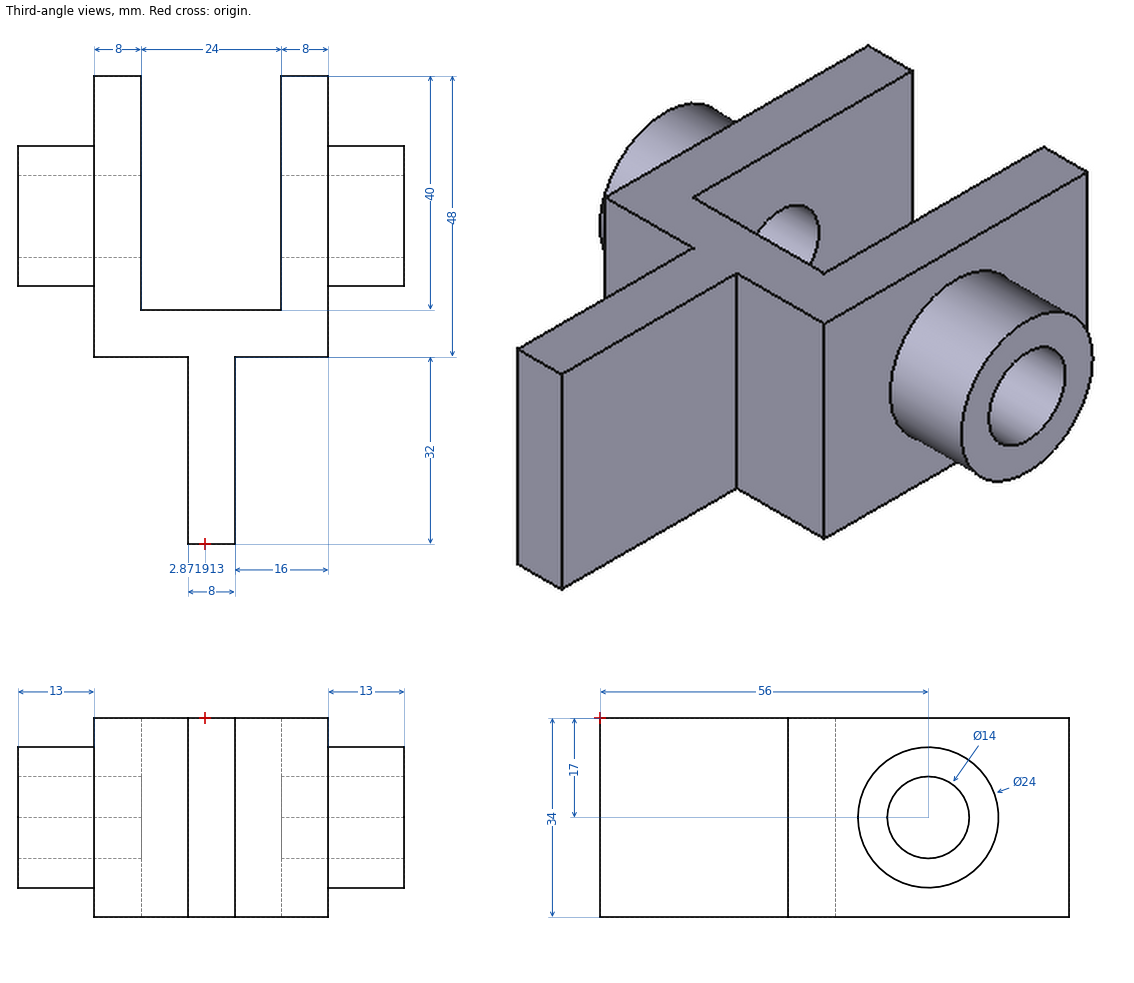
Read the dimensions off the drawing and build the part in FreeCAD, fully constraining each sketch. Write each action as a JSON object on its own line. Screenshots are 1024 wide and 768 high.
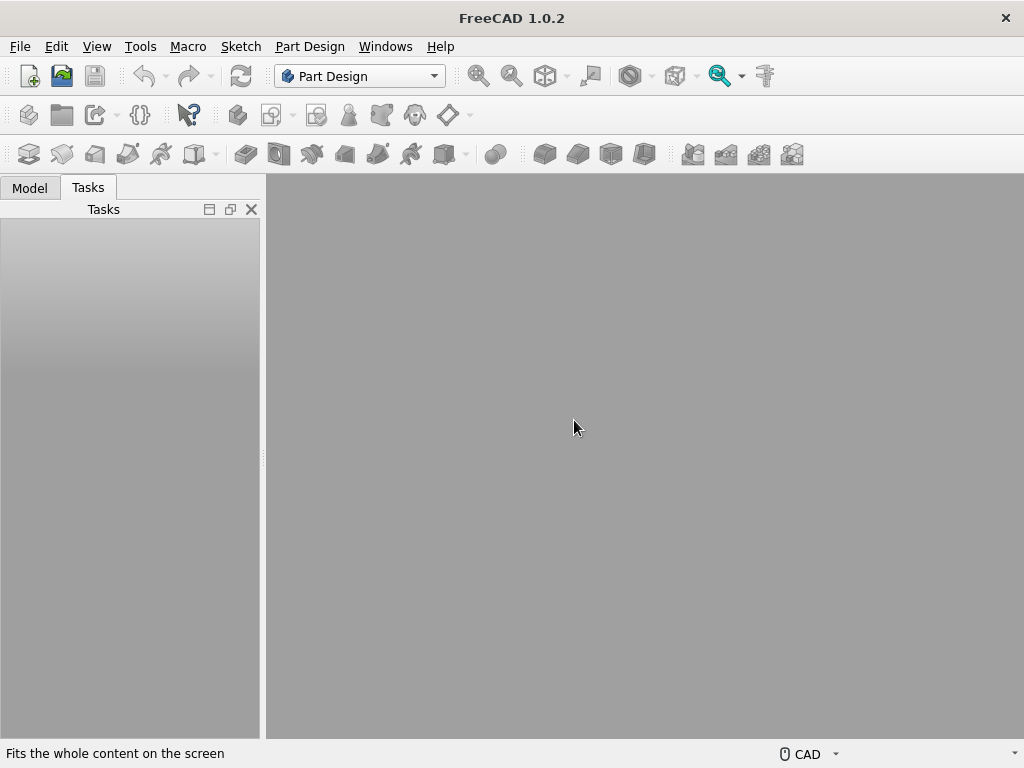
{"action": "key", "text": "ctrl+n"}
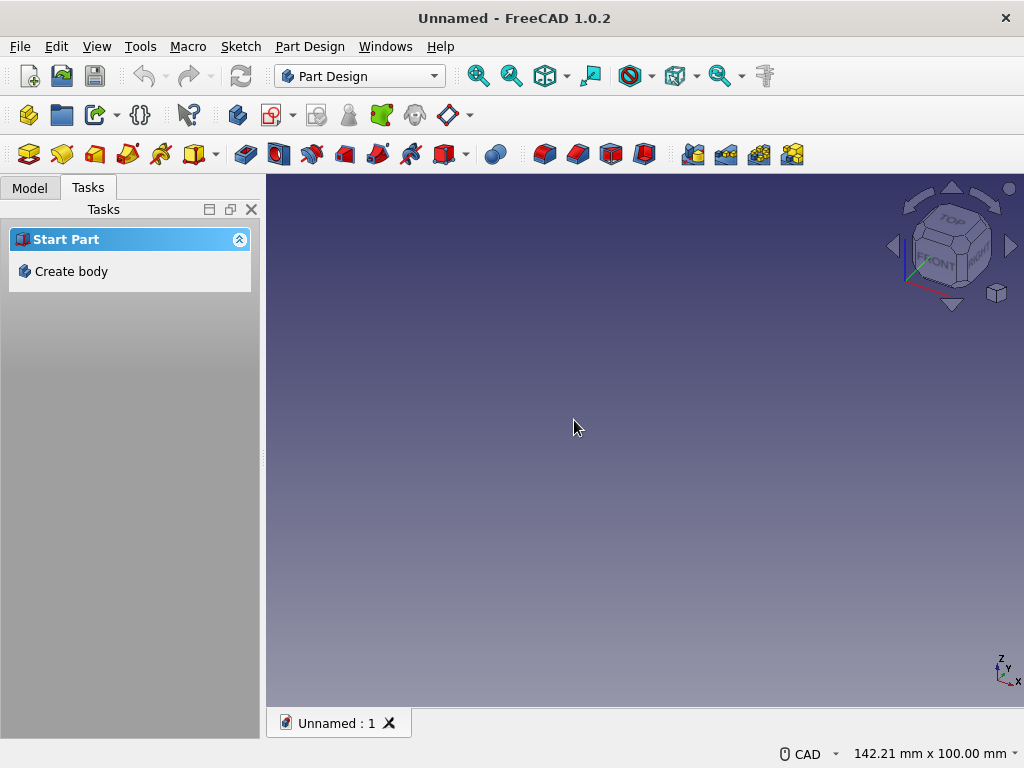
{"action": "left_click", "coordinate": [270, 116]}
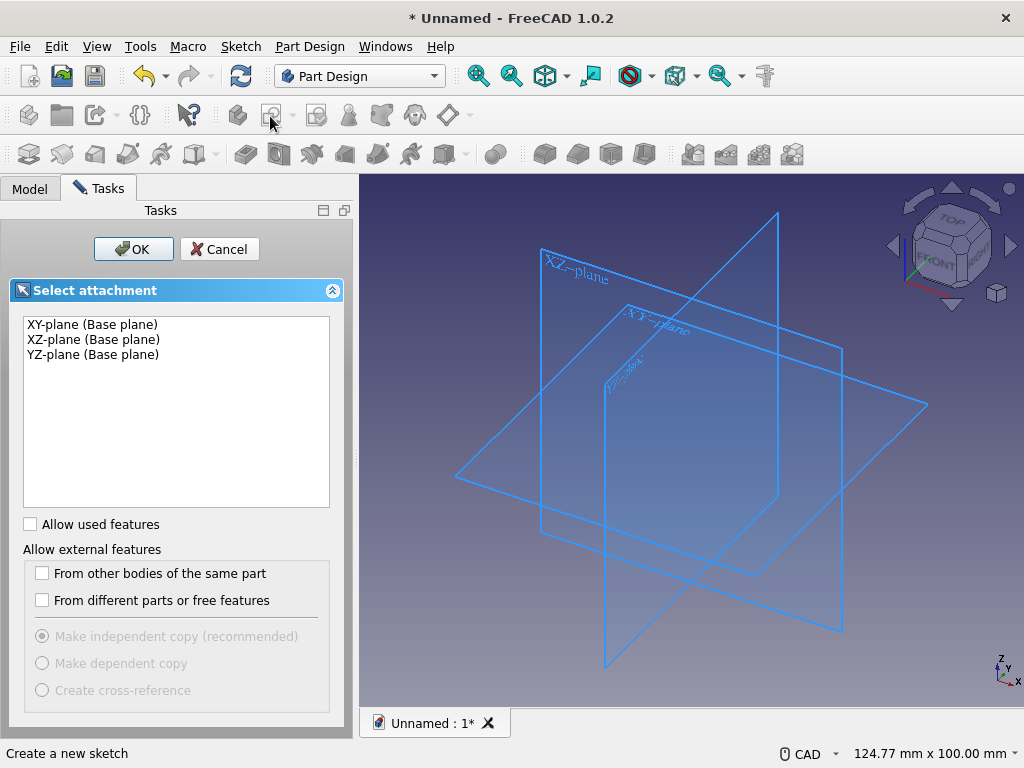
{"action": "left_click", "coordinate": [84, 324]}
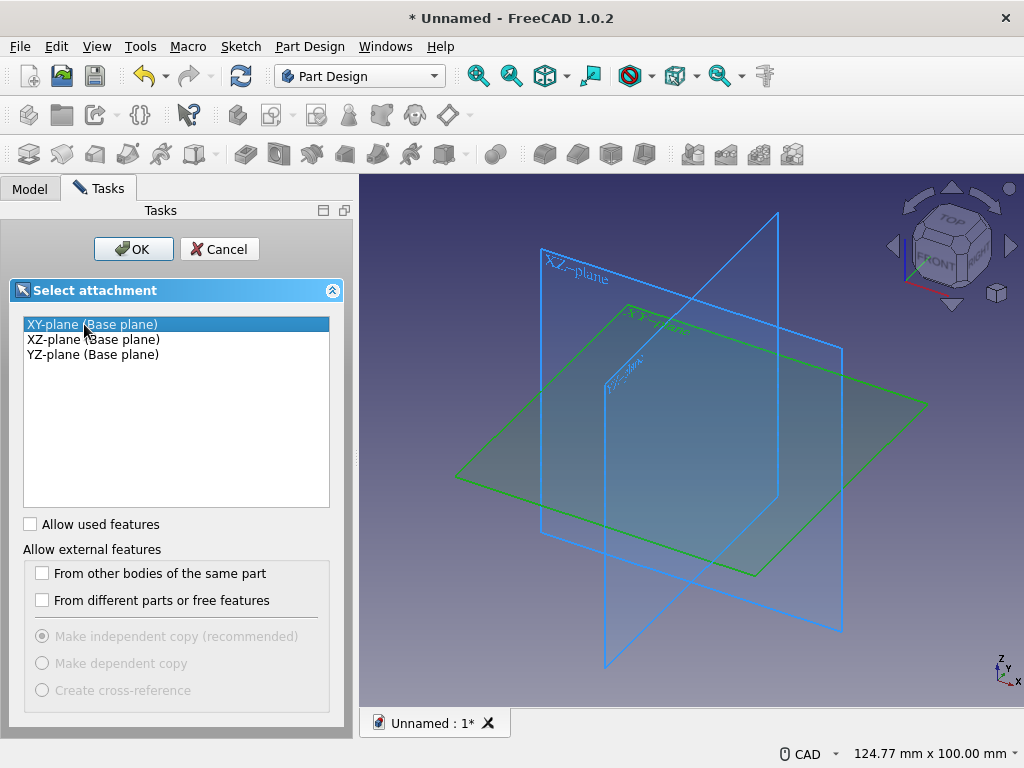
{"action": "left_click", "coordinate": [134, 249]}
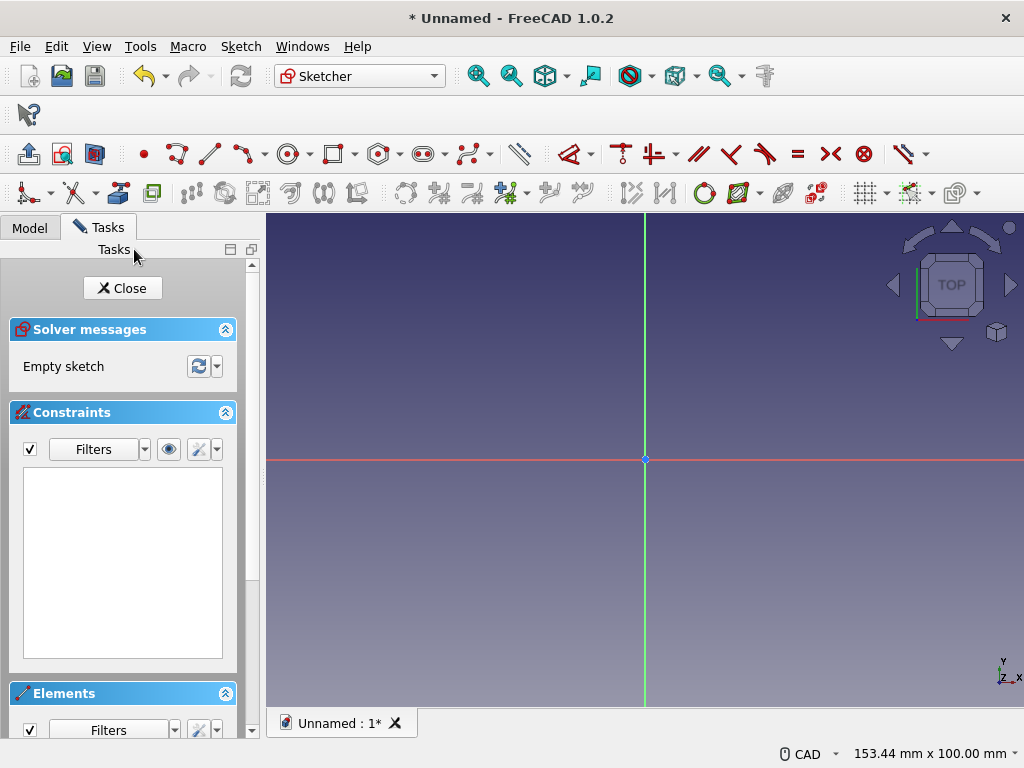
{"action": "scroll", "coordinate": [426, 679], "scroll_direction": "down", "scroll_amount": 2}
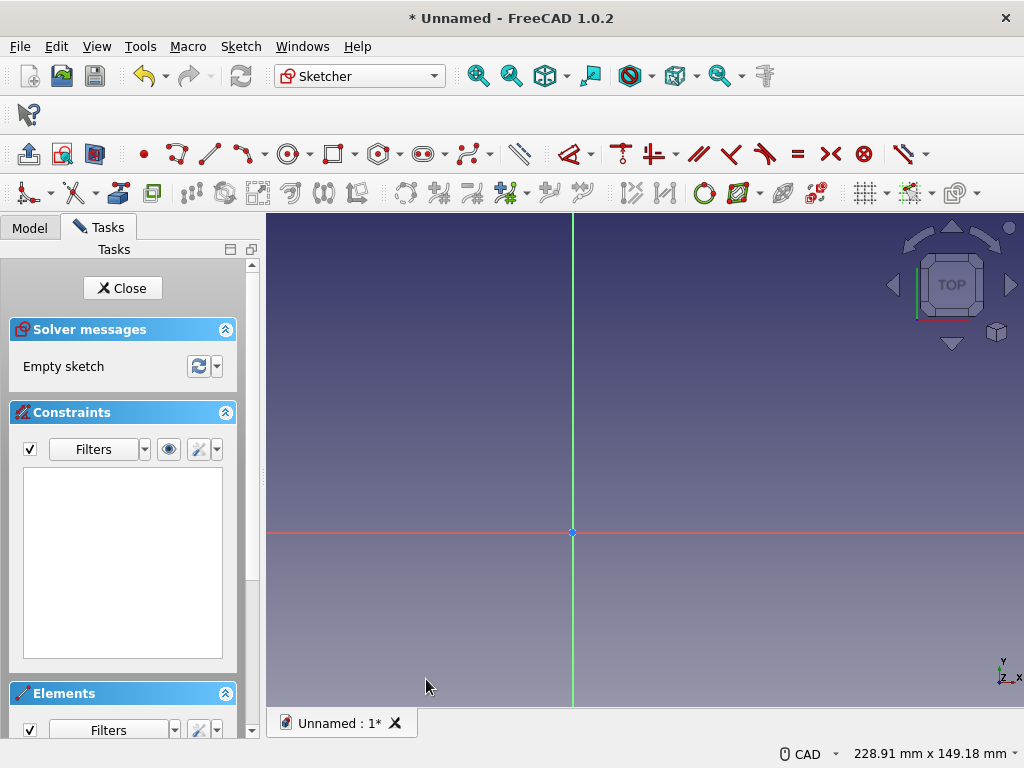
{"action": "left_click", "coordinate": [177, 154]}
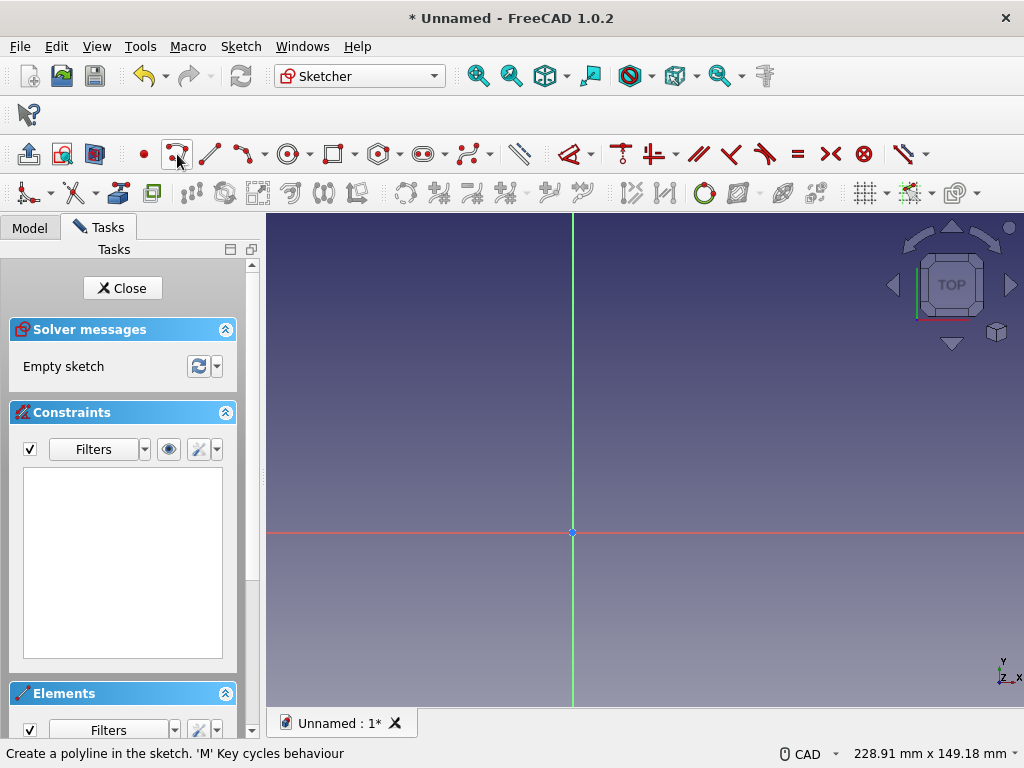
{"action": "scroll", "coordinate": [563, 533], "scroll_direction": "up", "scroll_amount": 3}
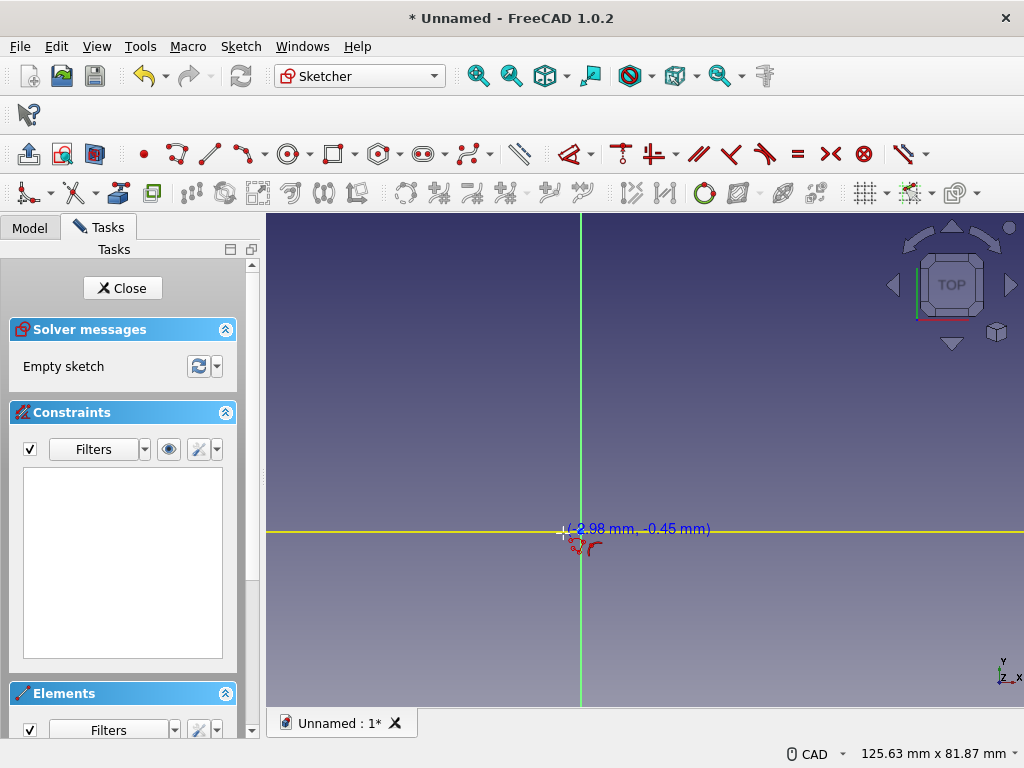
{"action": "left_click", "coordinate": [563, 532]}
{"action": "left_click", "coordinate": [612, 523]}
{"action": "left_click", "coordinate": [612, 338]}
{"action": "left_click", "coordinate": [708, 338]}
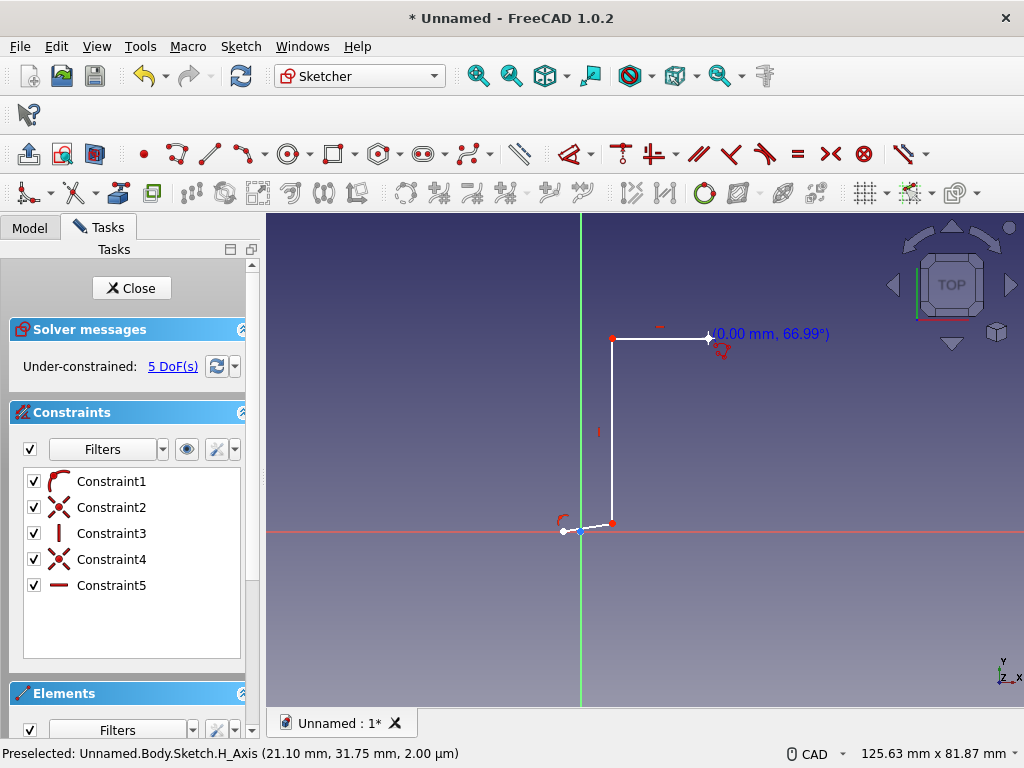
{"action": "scroll", "coordinate": [563, 667], "scroll_direction": "down", "scroll_amount": 3}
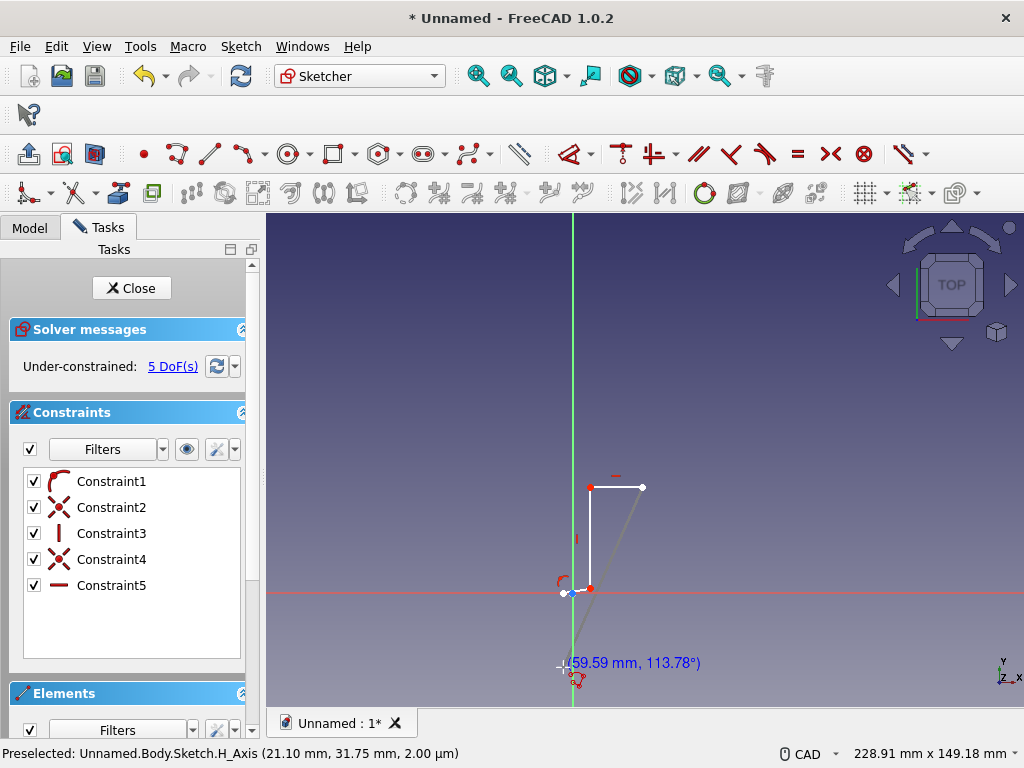
{"action": "left_click", "coordinate": [643, 328]}
{"action": "left_click", "coordinate": [616, 328]}
{"action": "left_click", "coordinate": [616, 461]}
{"action": "left_click", "coordinate": [537, 461]}
{"action": "left_click", "coordinate": [537, 328]}
{"action": "left_click", "coordinate": [510, 328]}
{"action": "left_click", "coordinate": [510, 487]}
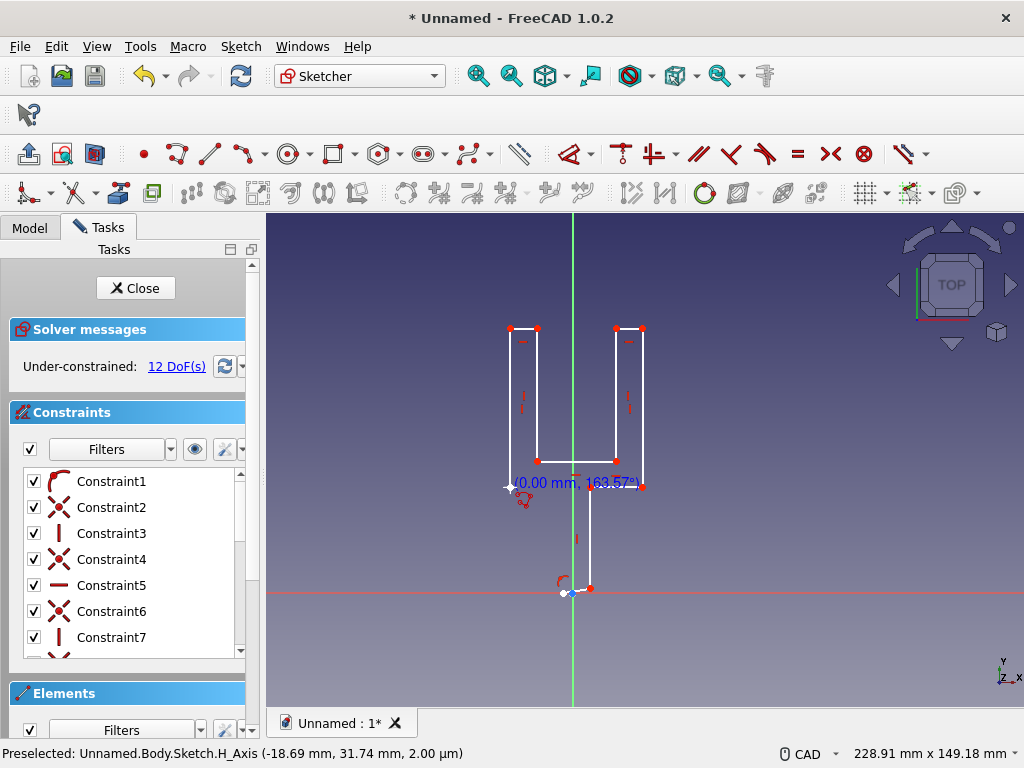
{"action": "scroll", "coordinate": [563, 487], "scroll_direction": "up", "scroll_amount": 3}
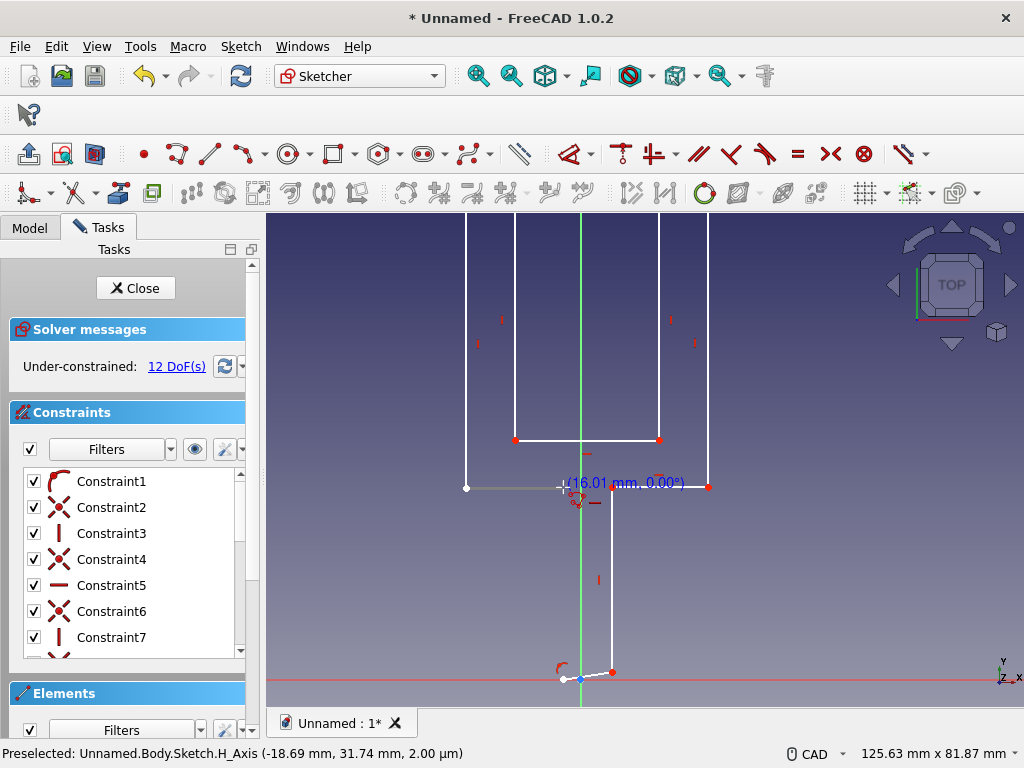
{"action": "left_click", "coordinate": [563, 487]}